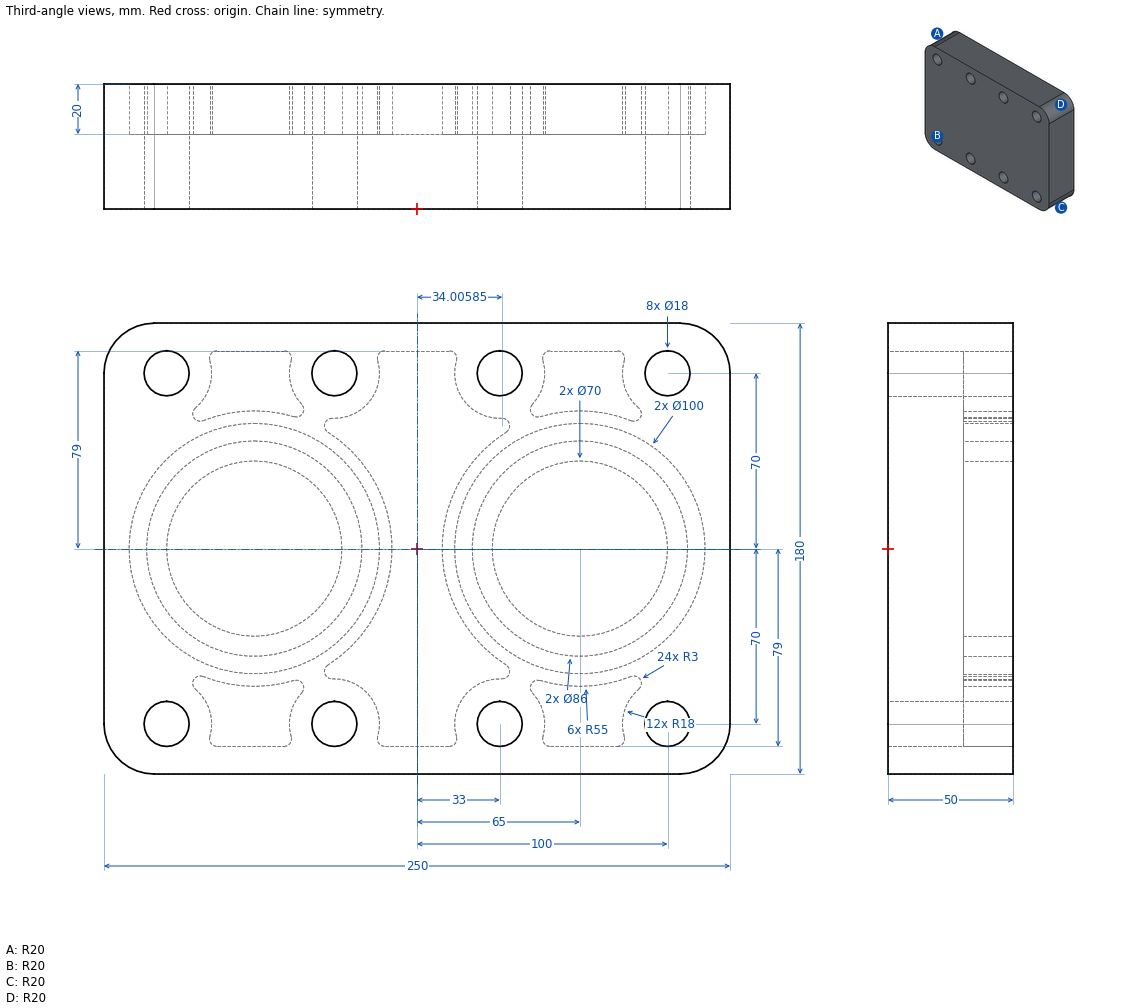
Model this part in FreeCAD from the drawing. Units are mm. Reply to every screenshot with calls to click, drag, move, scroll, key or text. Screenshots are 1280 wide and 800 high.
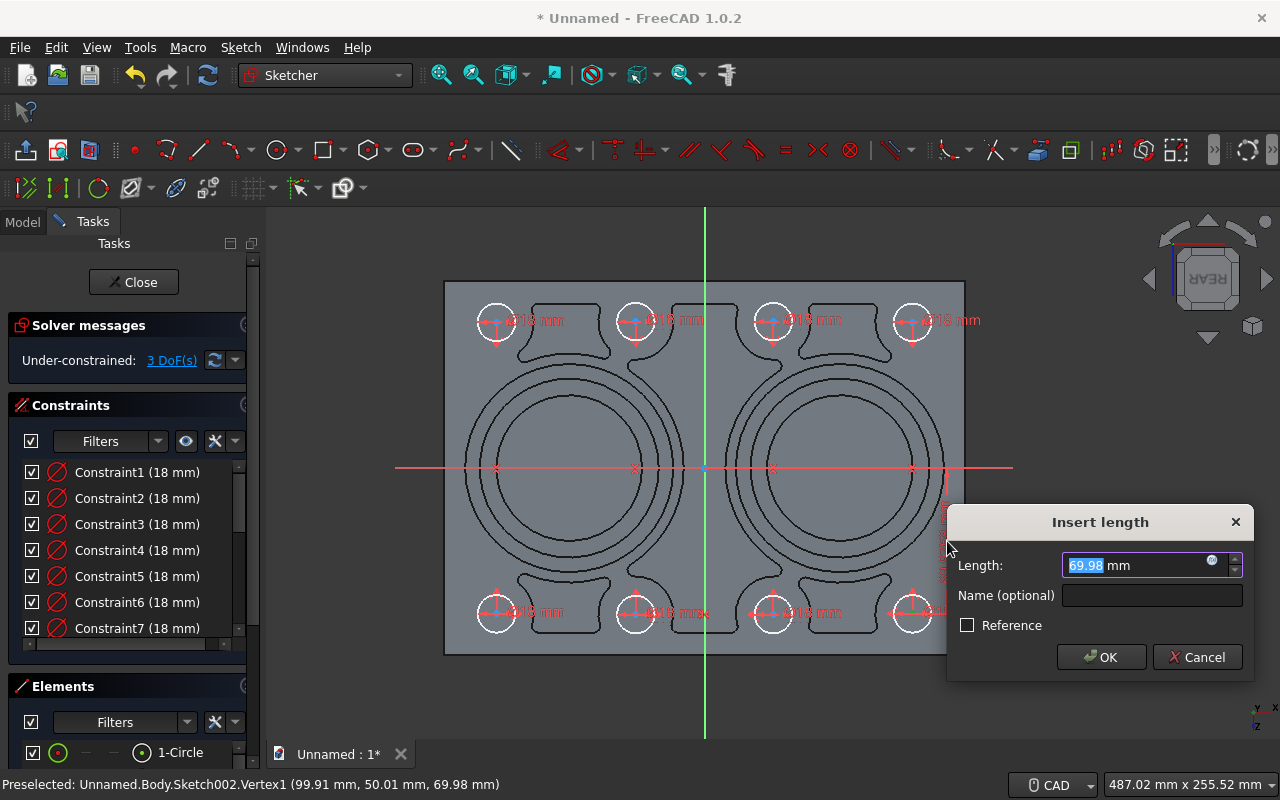
text(70)
key(Return)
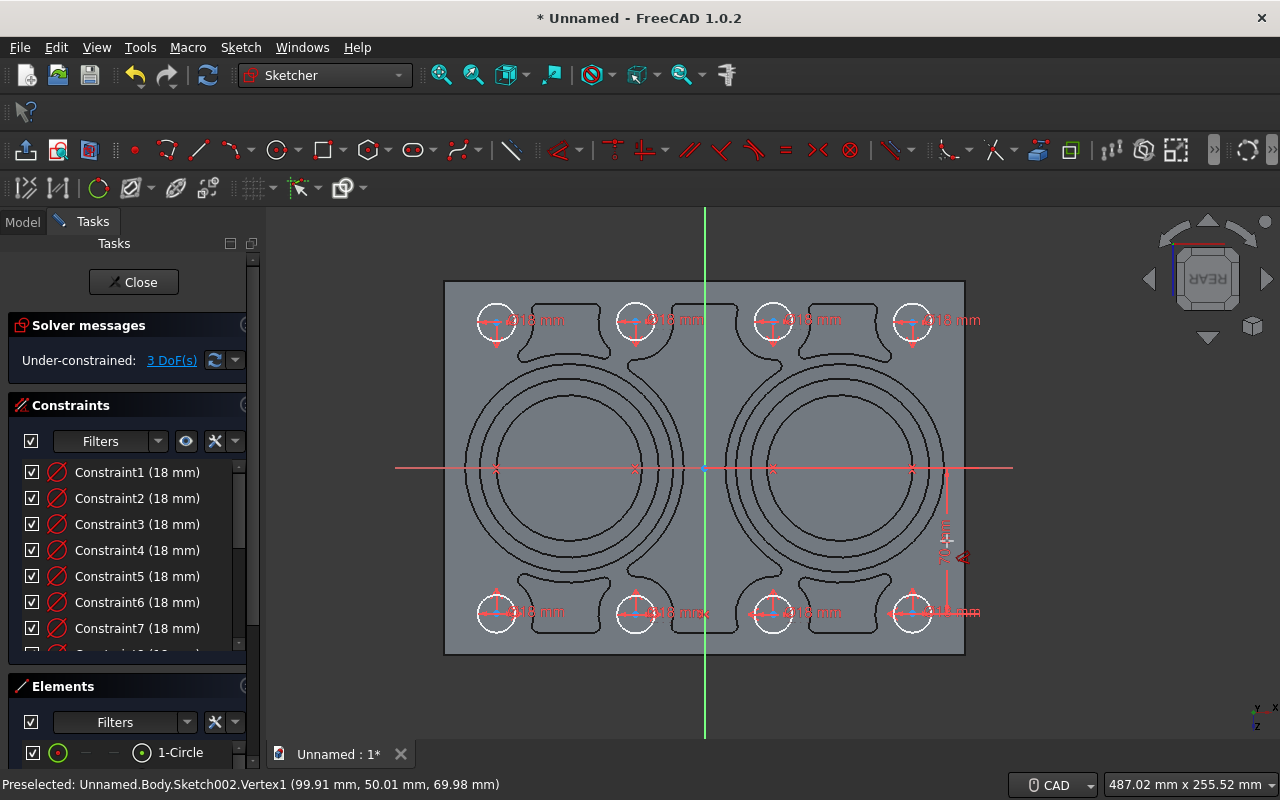
click(773, 615)
click(739, 649)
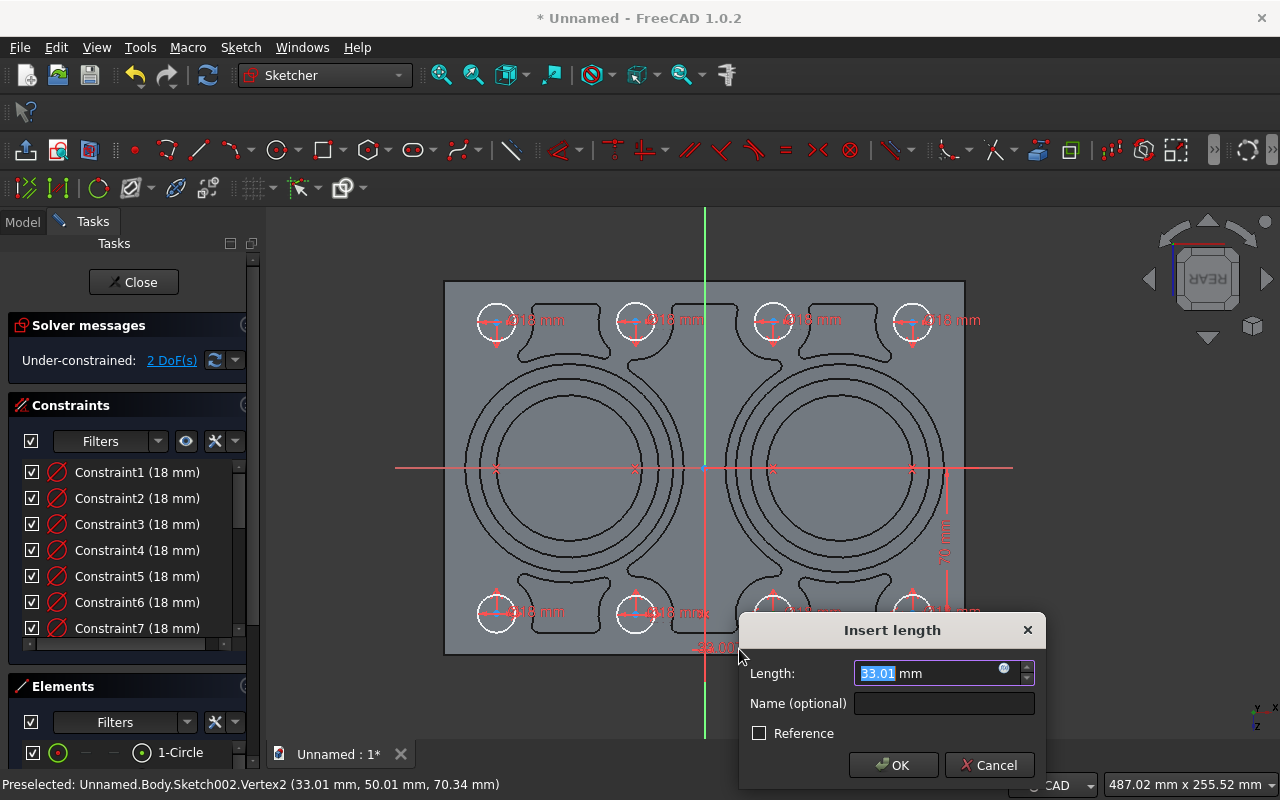
text(33)
key(Return)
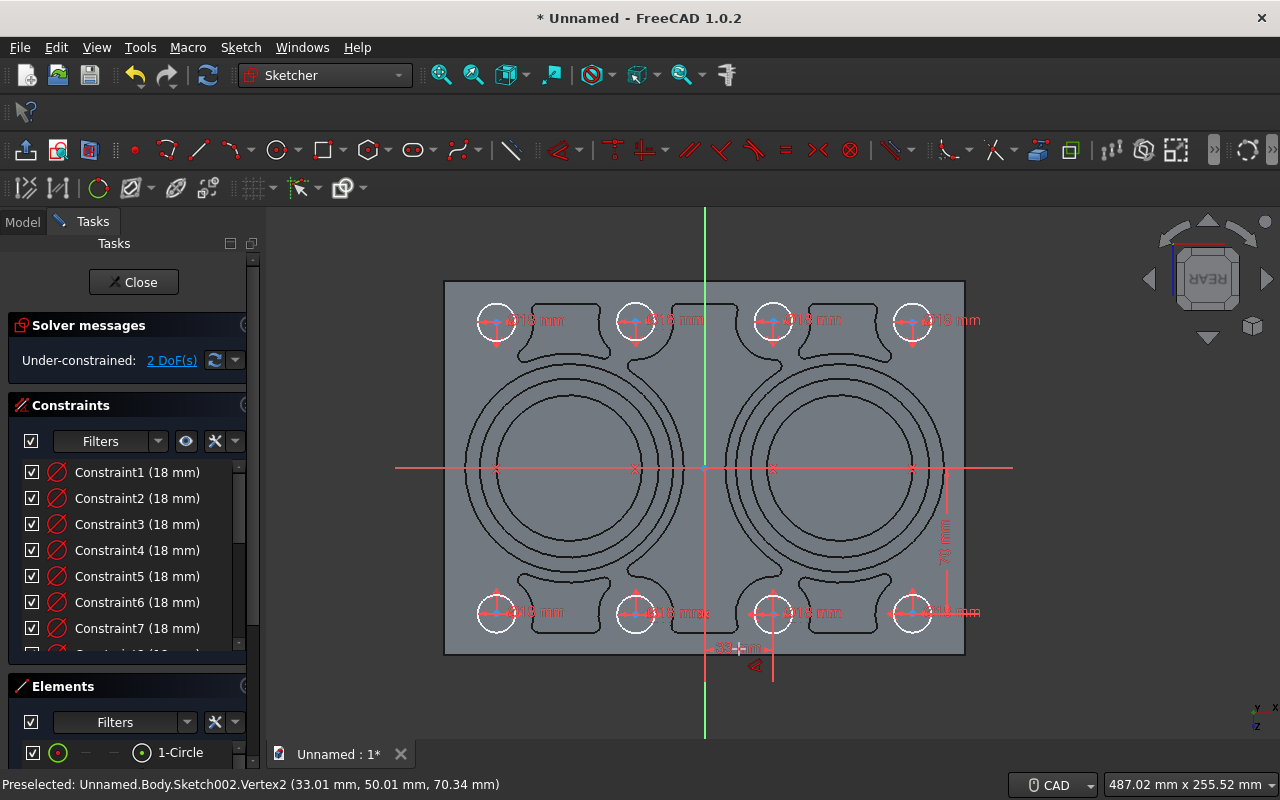
click(773, 615)
click(807, 541)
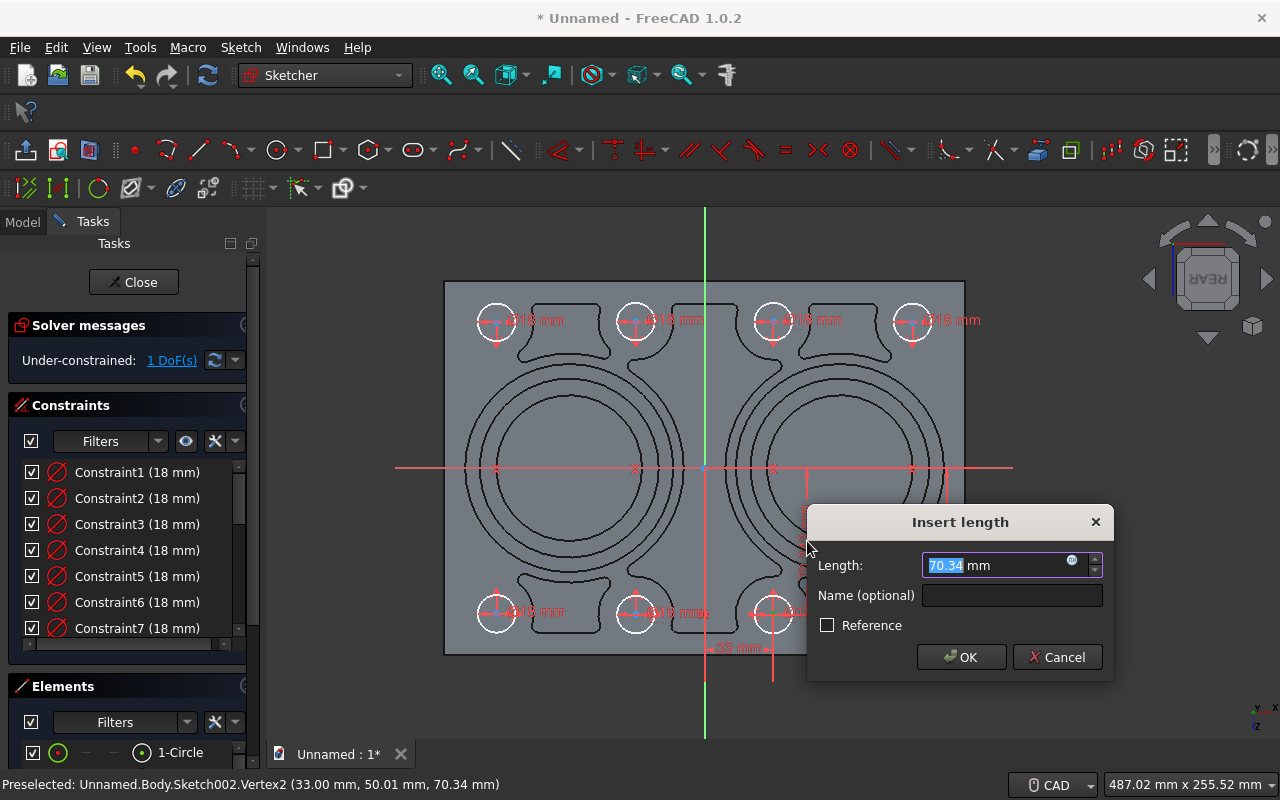
text(70)
key(Return)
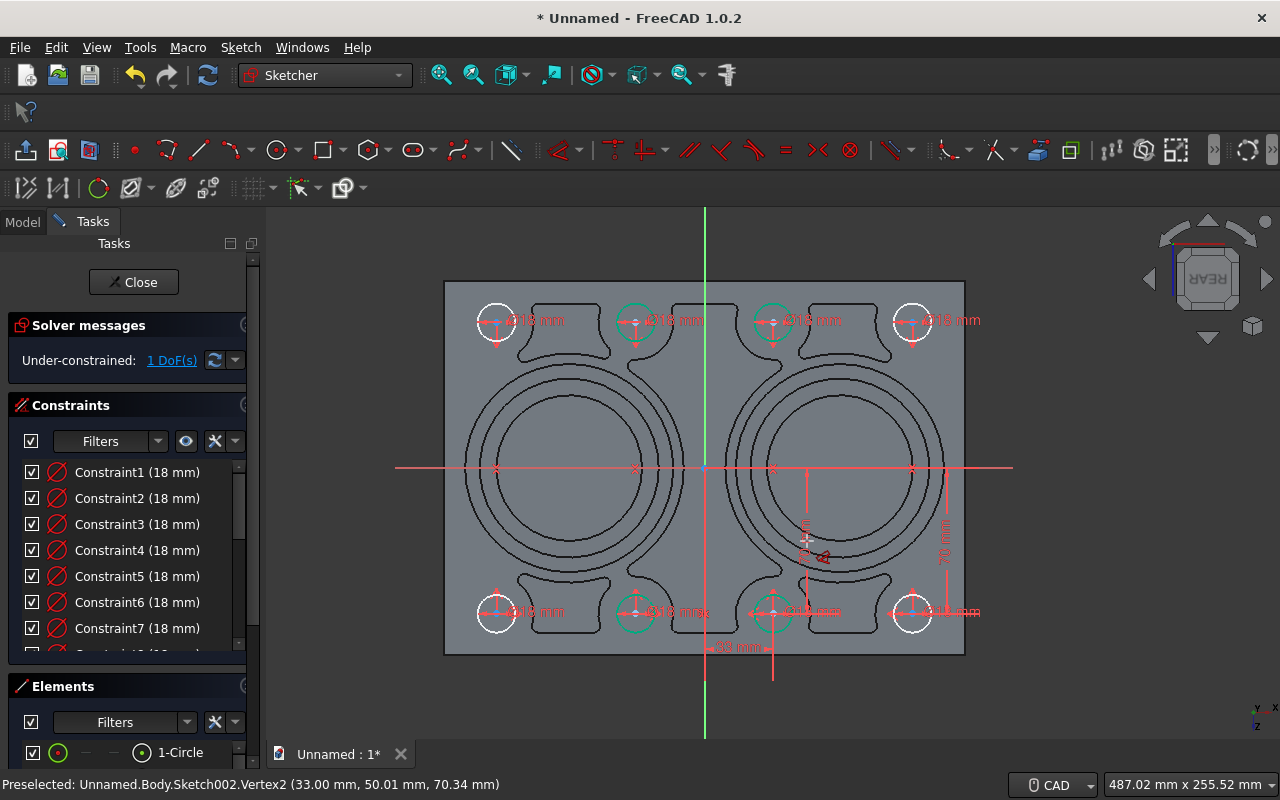
click(913, 614)
click(856, 648)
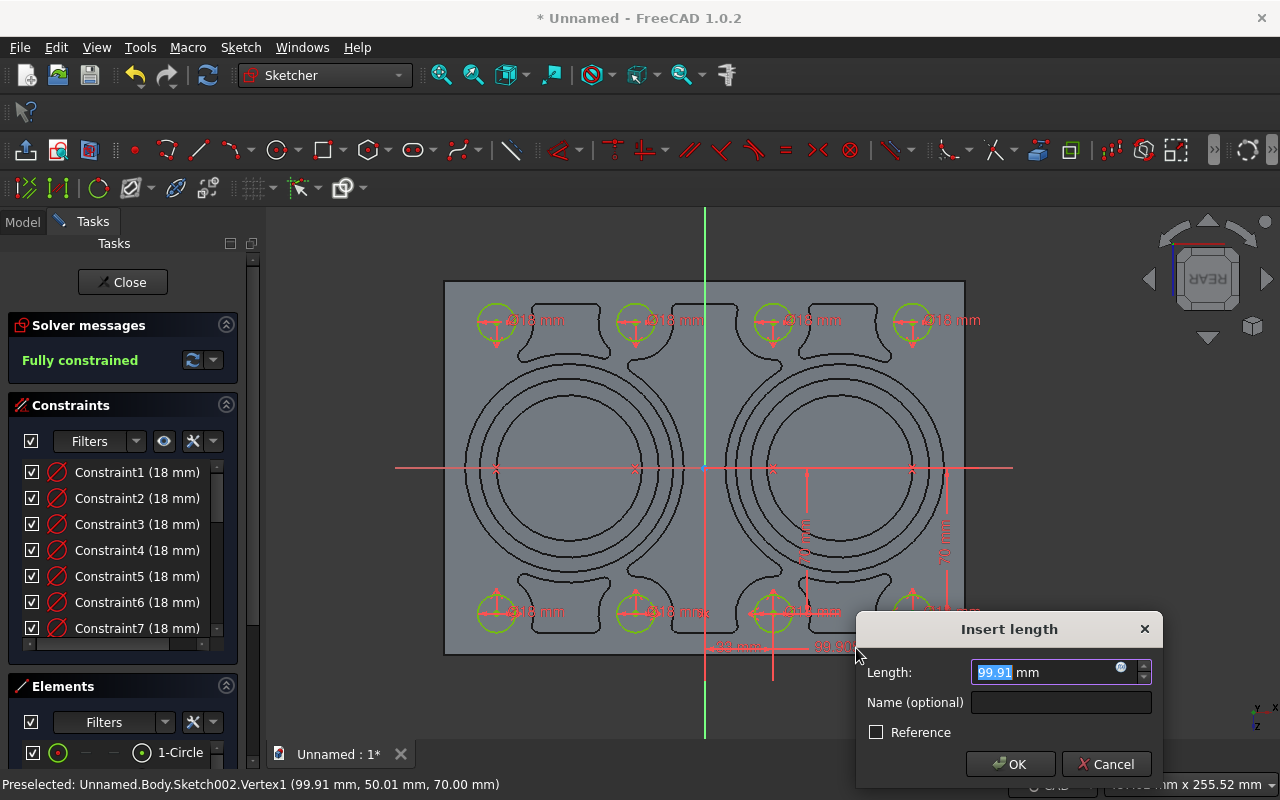
text(100)
key(Return)
key(Escape)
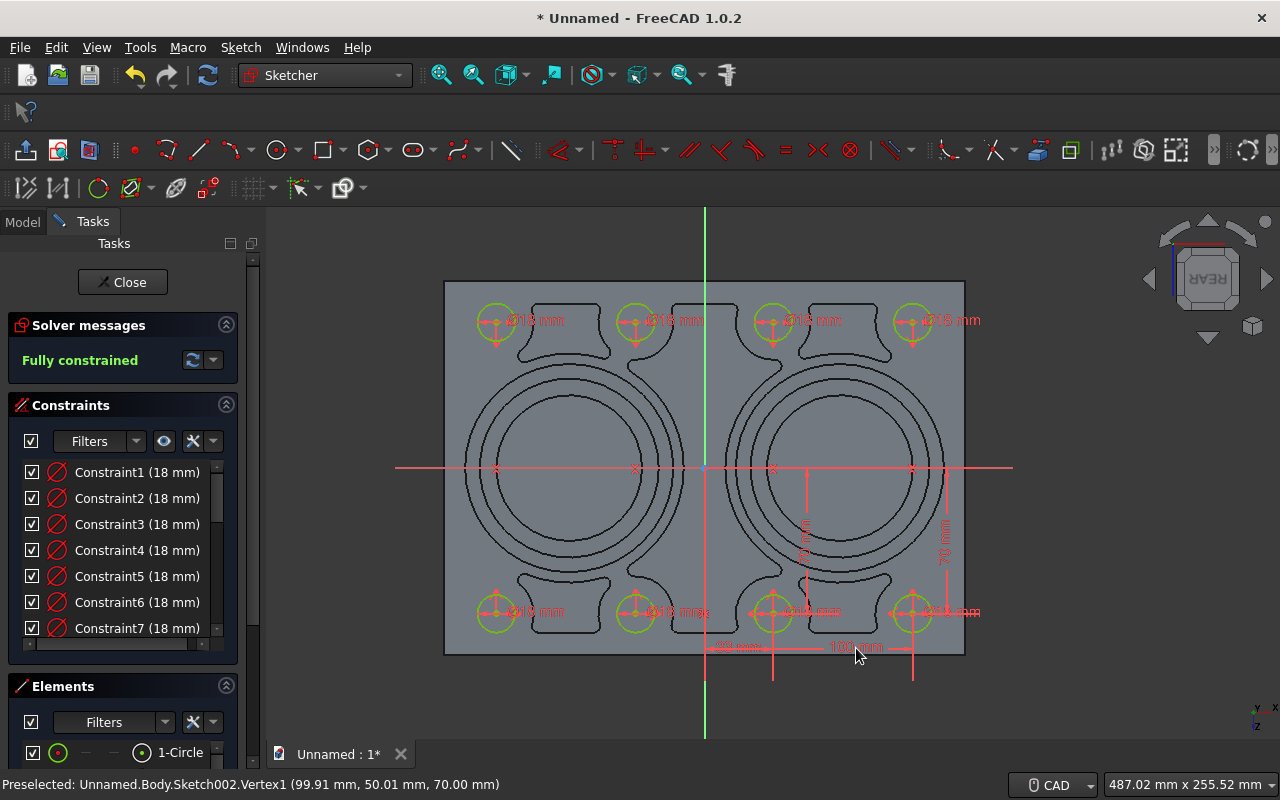
click(123, 282)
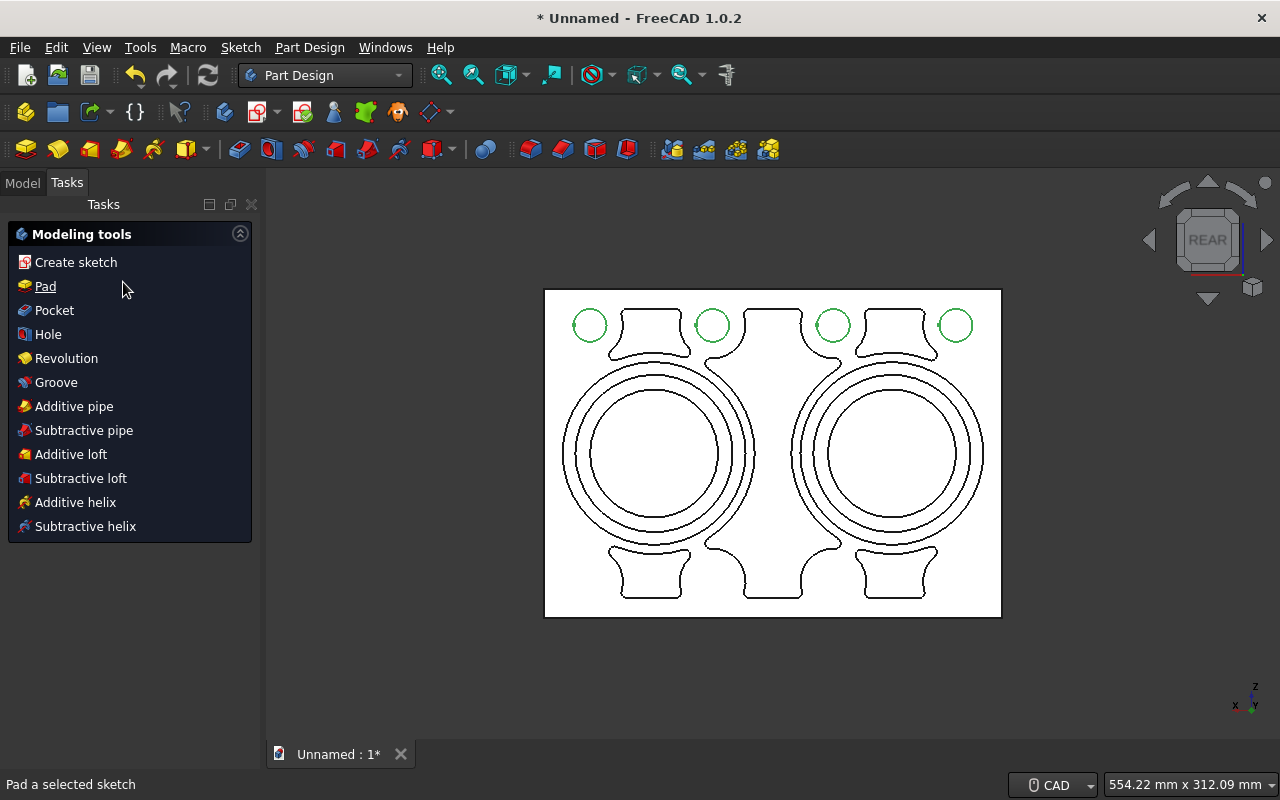
click(240, 150)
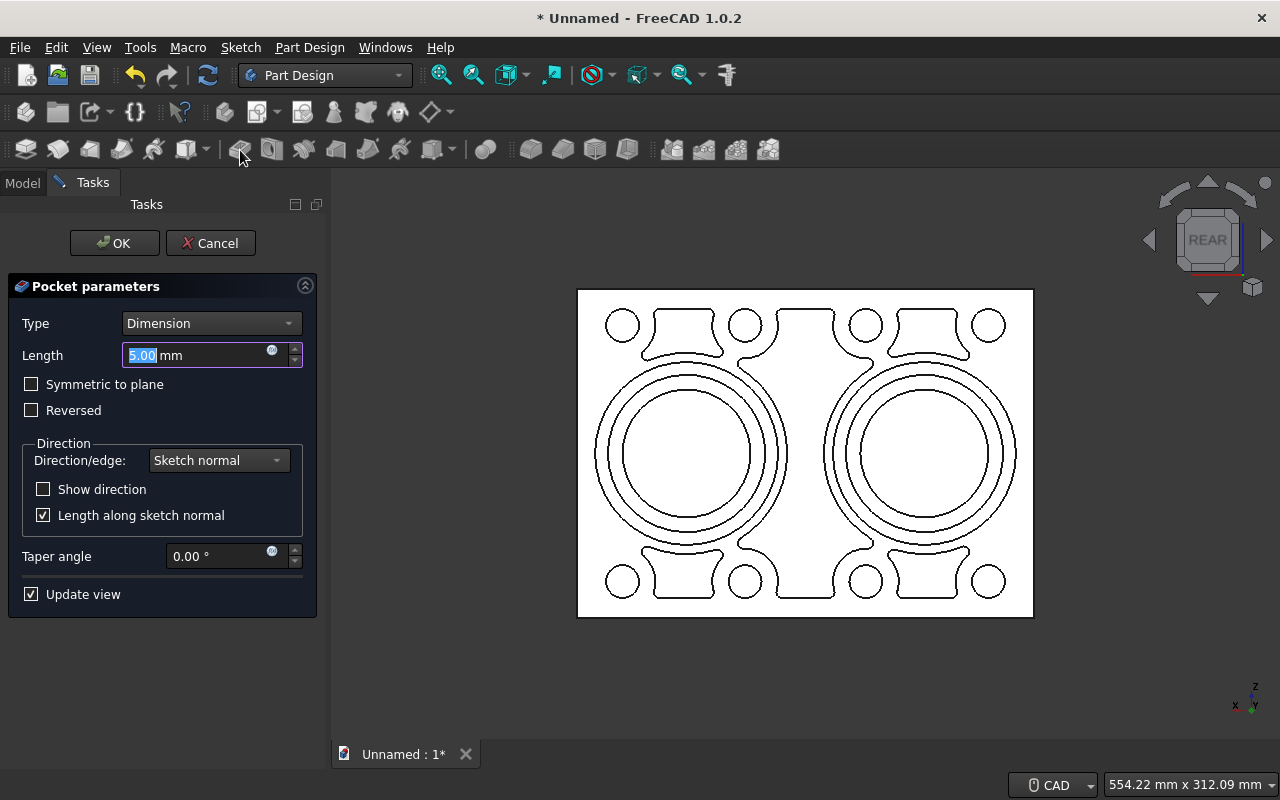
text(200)
key(Tab)